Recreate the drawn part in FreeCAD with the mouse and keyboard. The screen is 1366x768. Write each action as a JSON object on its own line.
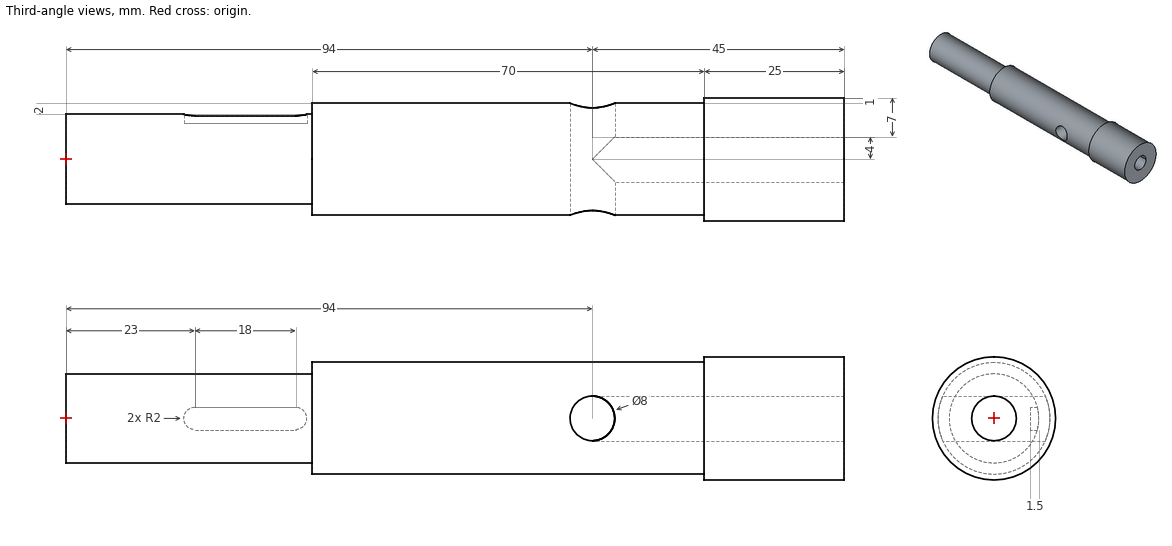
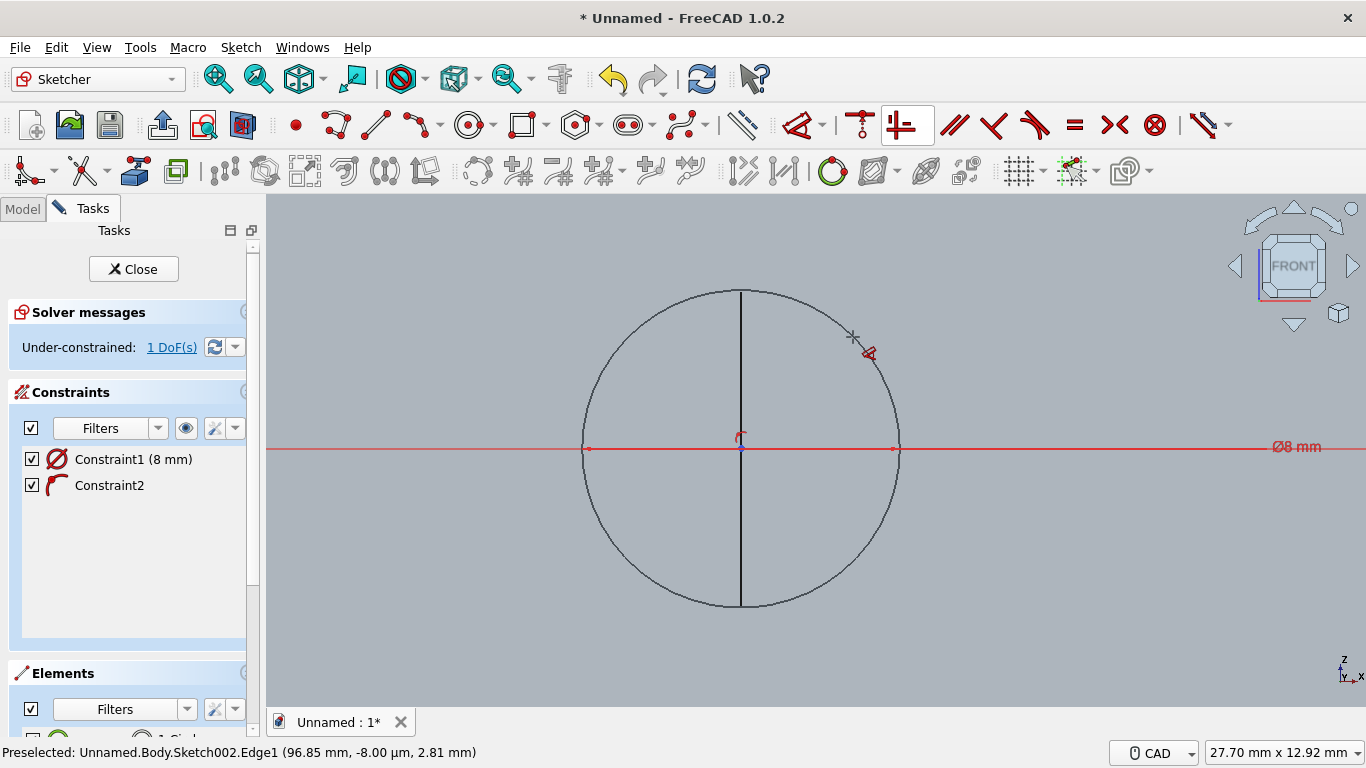
{"action": "left_click", "coordinate": [741, 449]}
{"action": "left_click", "coordinate": [518, 483]}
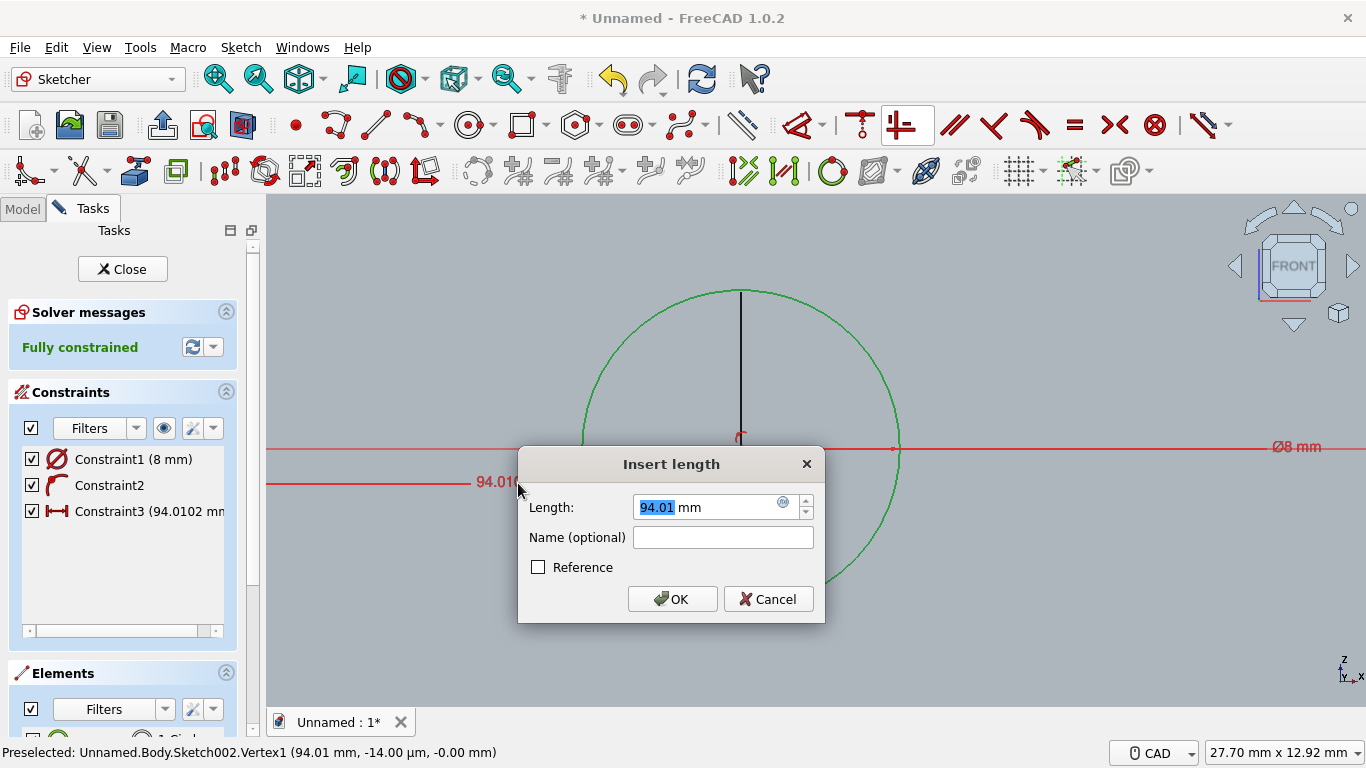
{"action": "type", "text": "94"}
{"action": "key", "text": "Return"}
{"action": "key", "text": "Escape"}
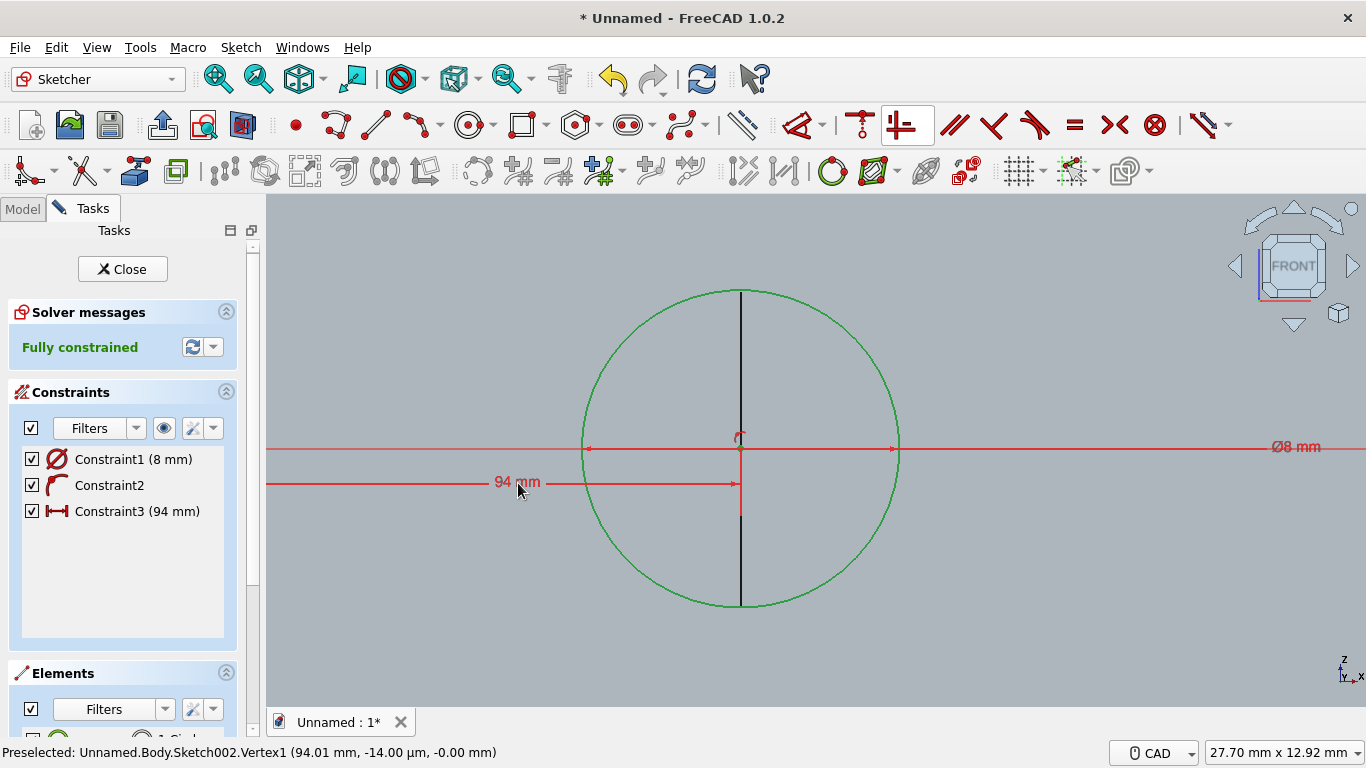
{"action": "left_click", "coordinate": [123, 269]}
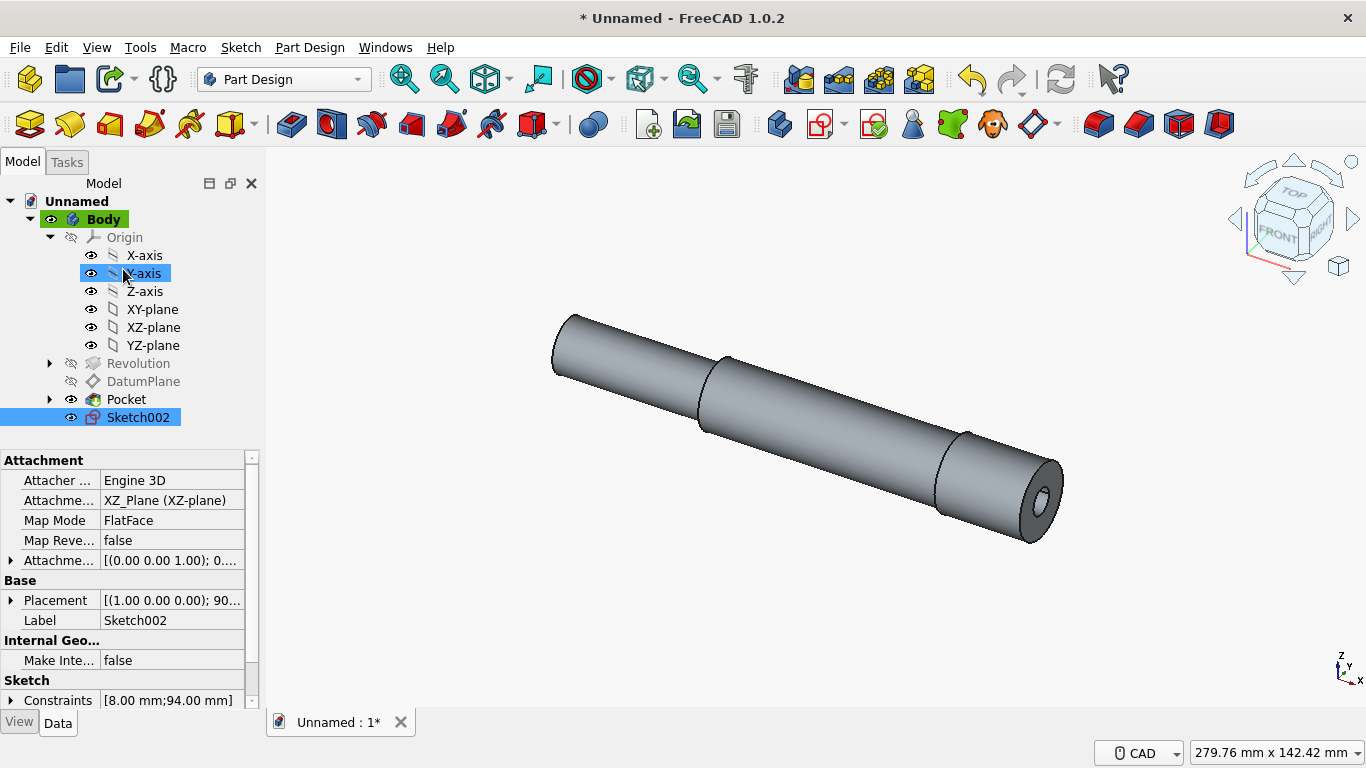
{"action": "left_click", "coordinate": [292, 124]}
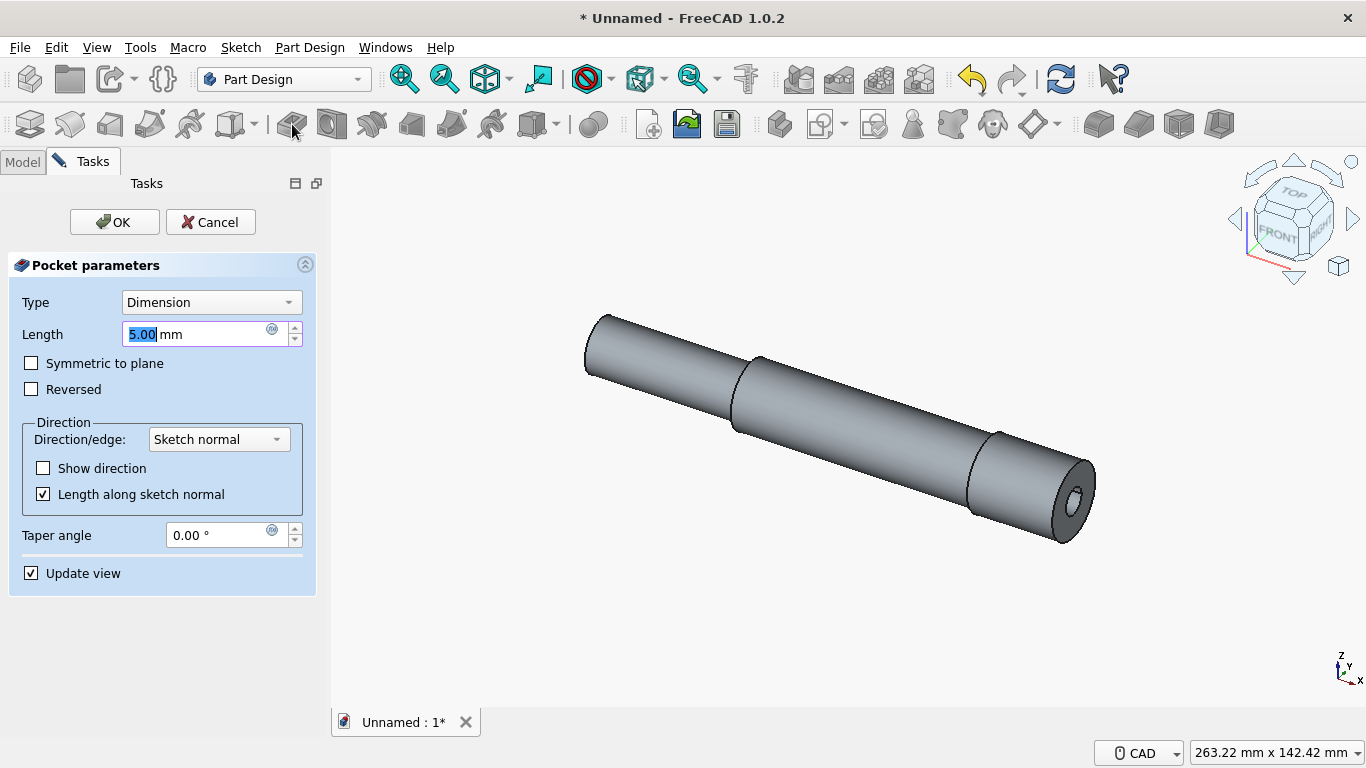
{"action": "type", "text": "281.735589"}
{"action": "key", "text": "Tab"}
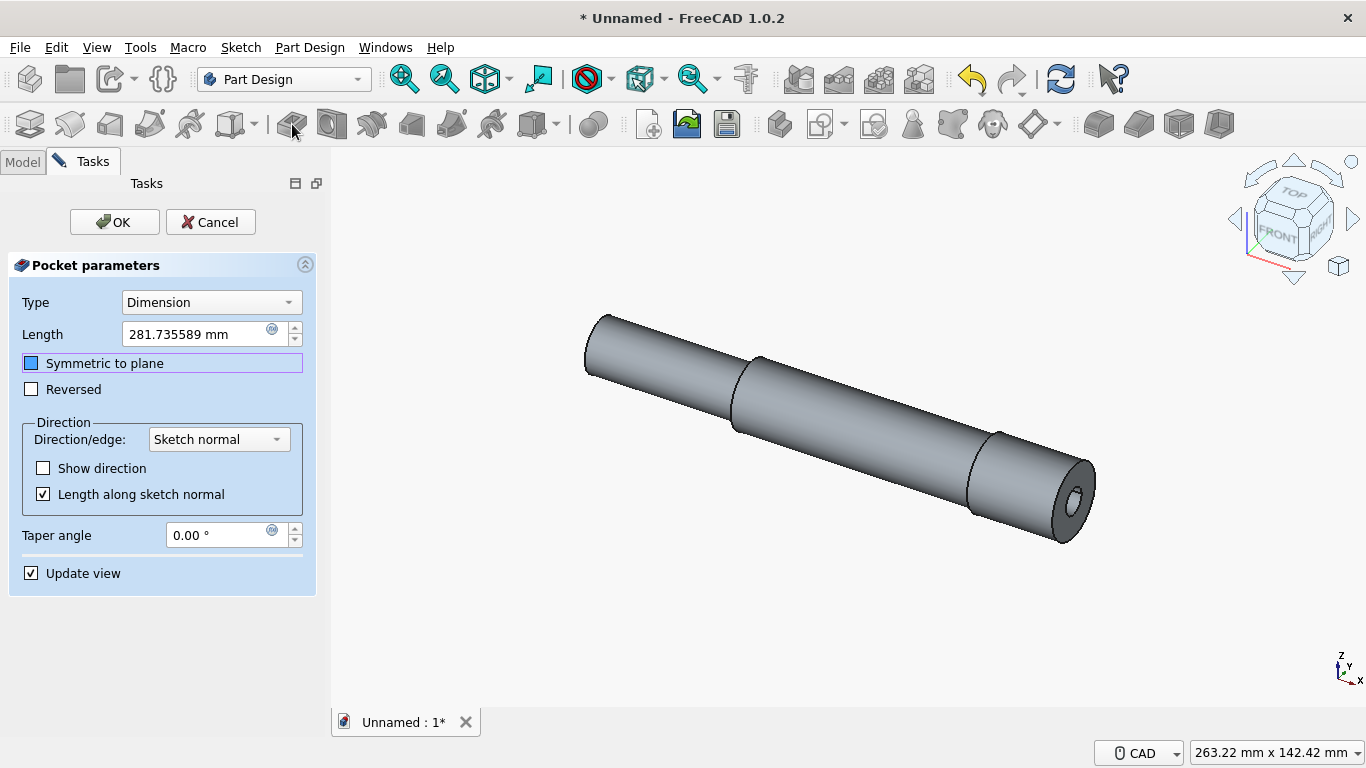
{"action": "left_click", "coordinate": [30, 363]}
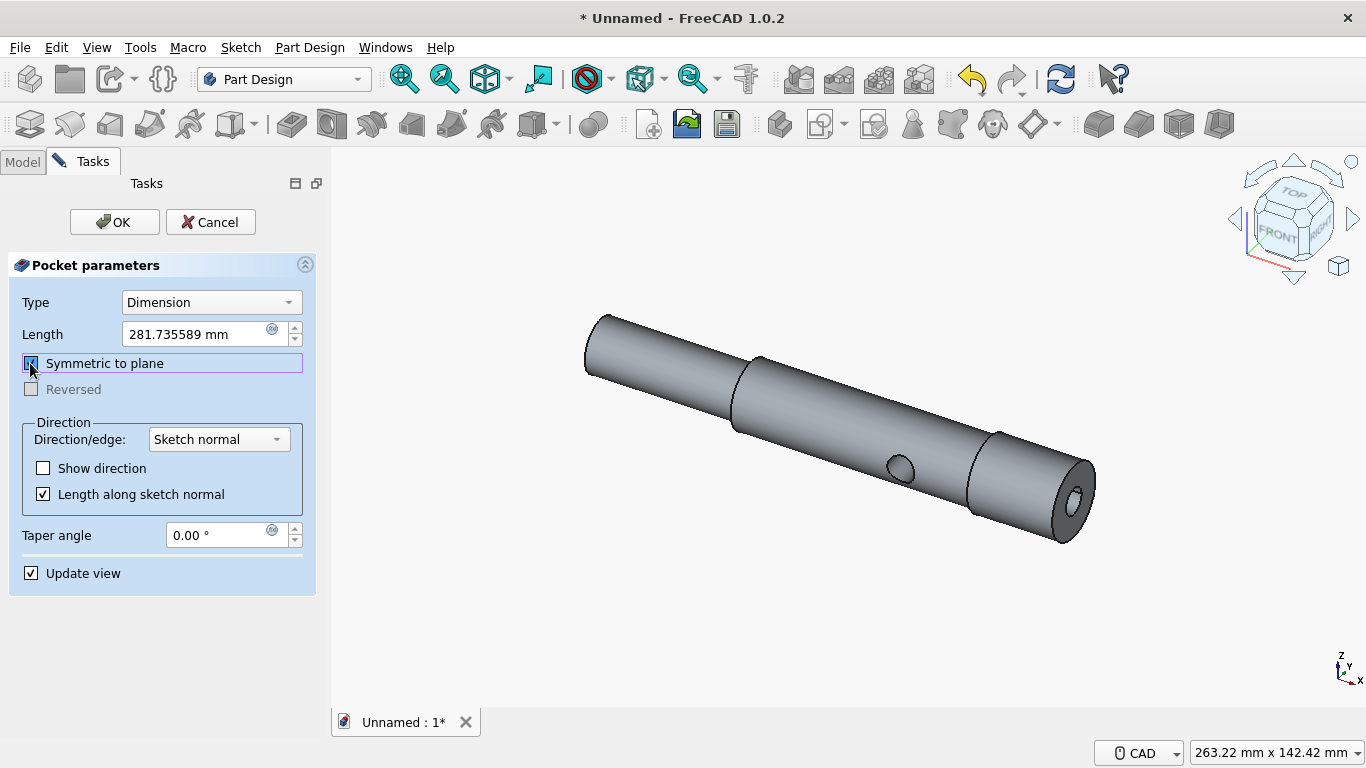
{"action": "left_click", "coordinate": [115, 222]}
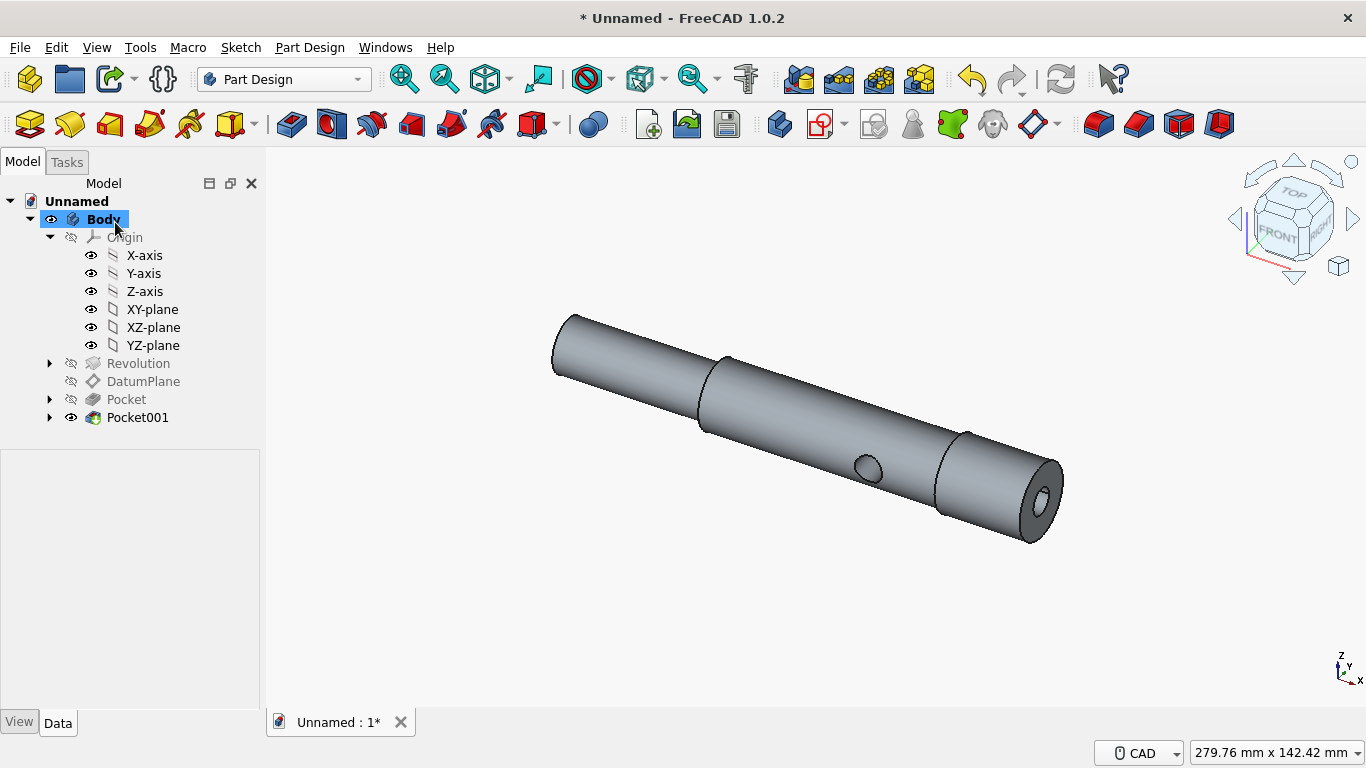
{"action": "key", "text": "0"}